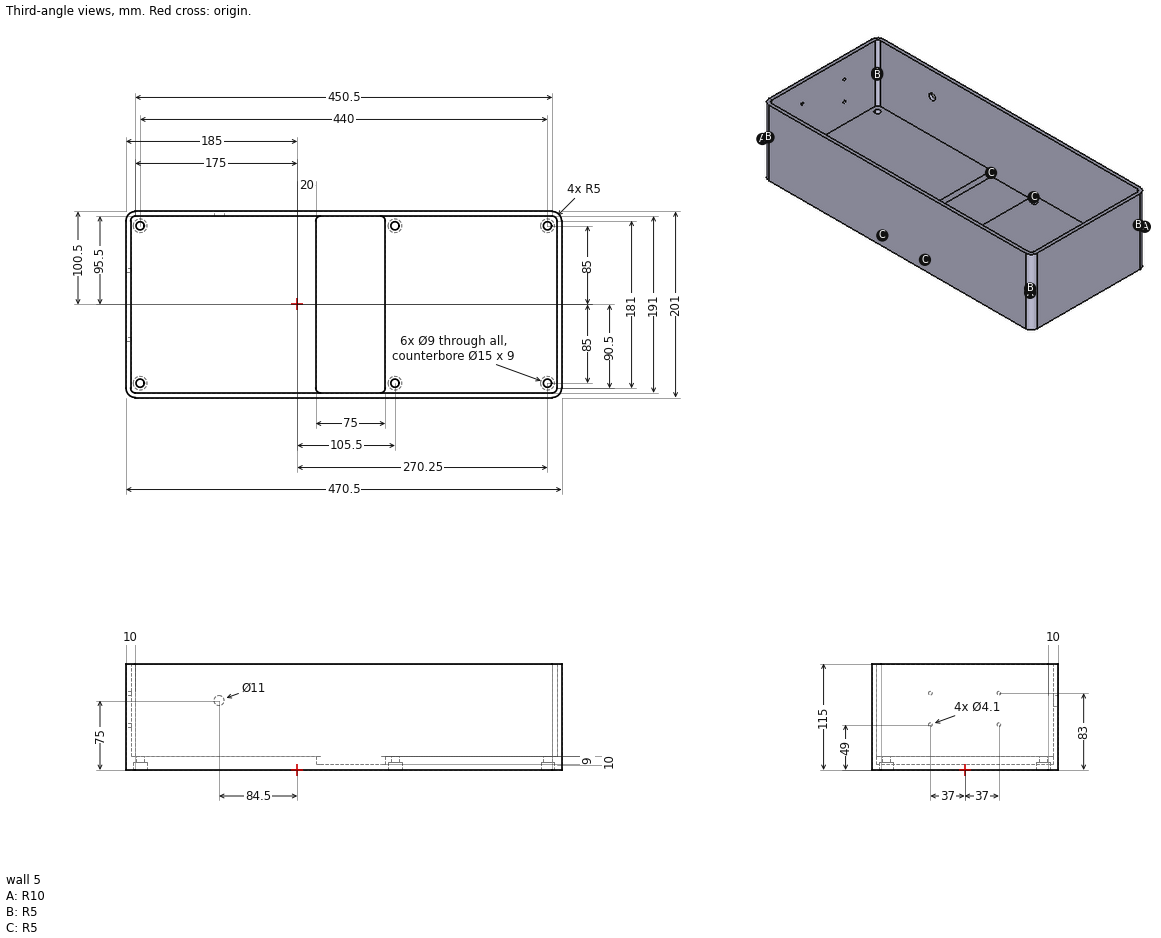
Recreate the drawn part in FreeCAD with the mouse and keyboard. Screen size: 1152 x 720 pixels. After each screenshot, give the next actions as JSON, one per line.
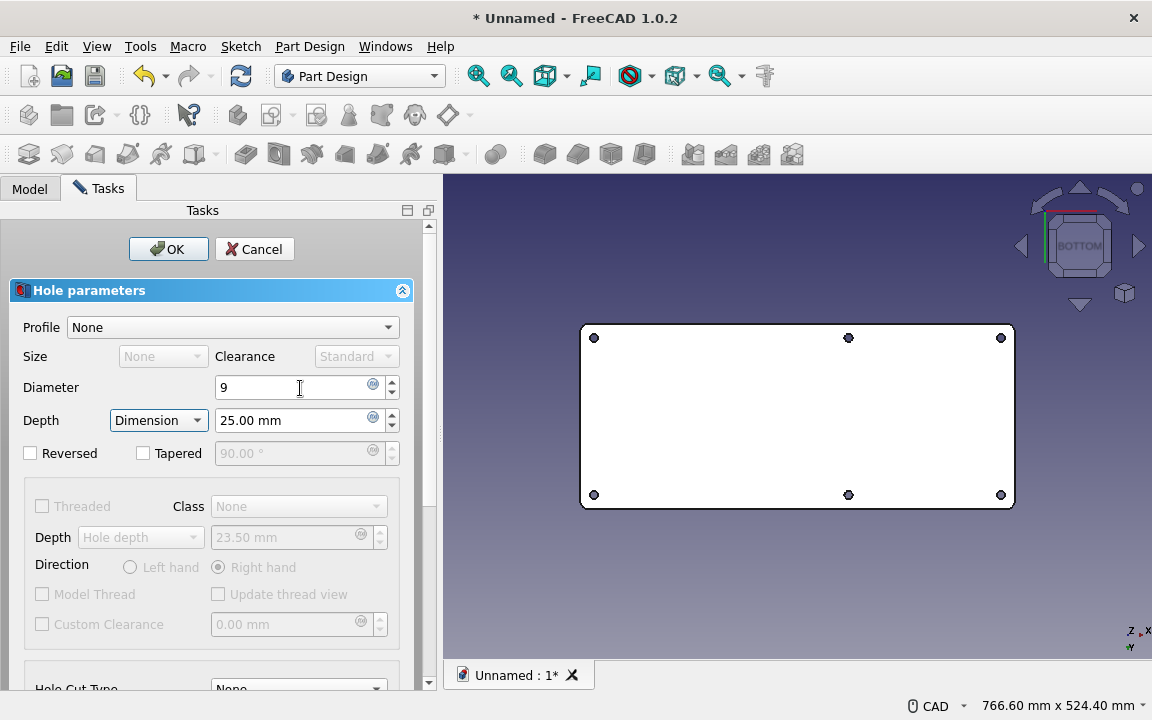
{"action": "left_click", "coordinate": [160, 420]}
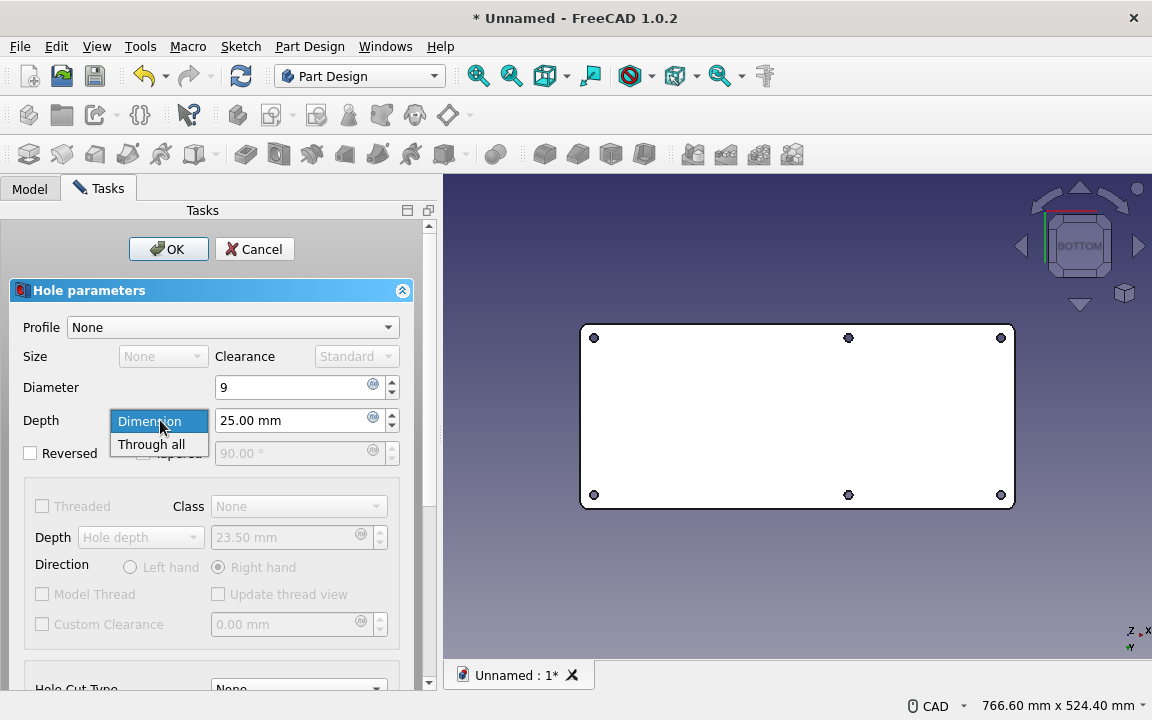
{"action": "left_click", "coordinate": [158, 444]}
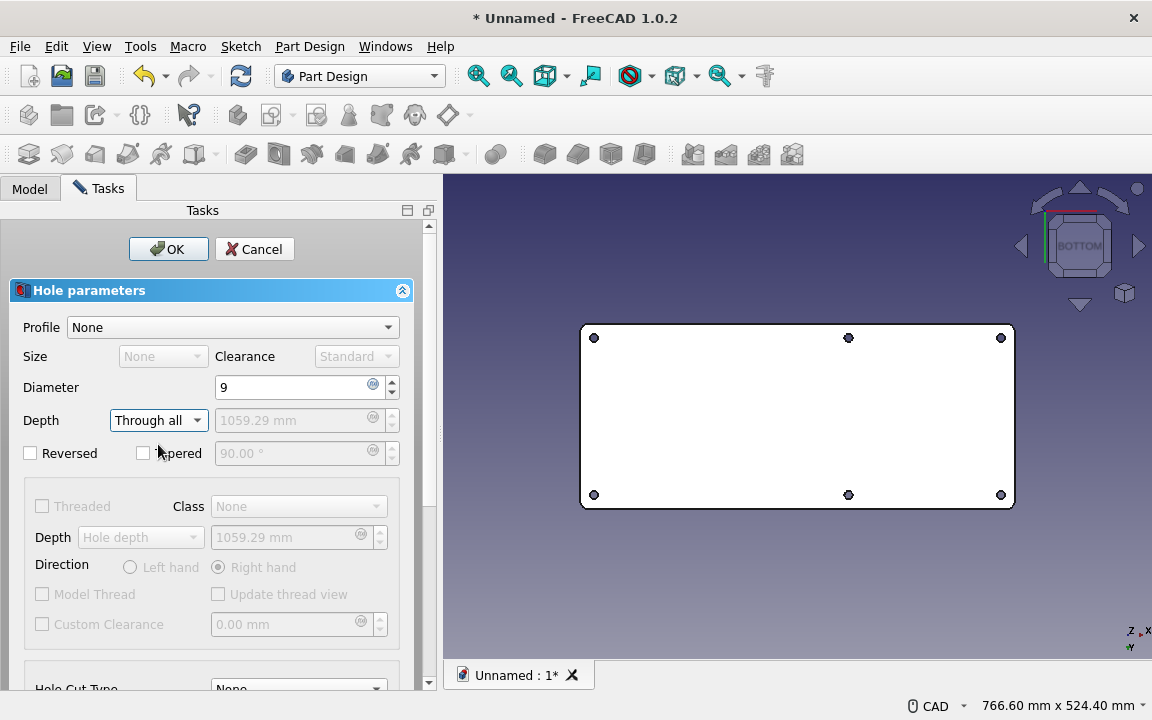
{"action": "scroll", "coordinate": [429, 455], "scroll_direction": "down", "scroll_amount": 2}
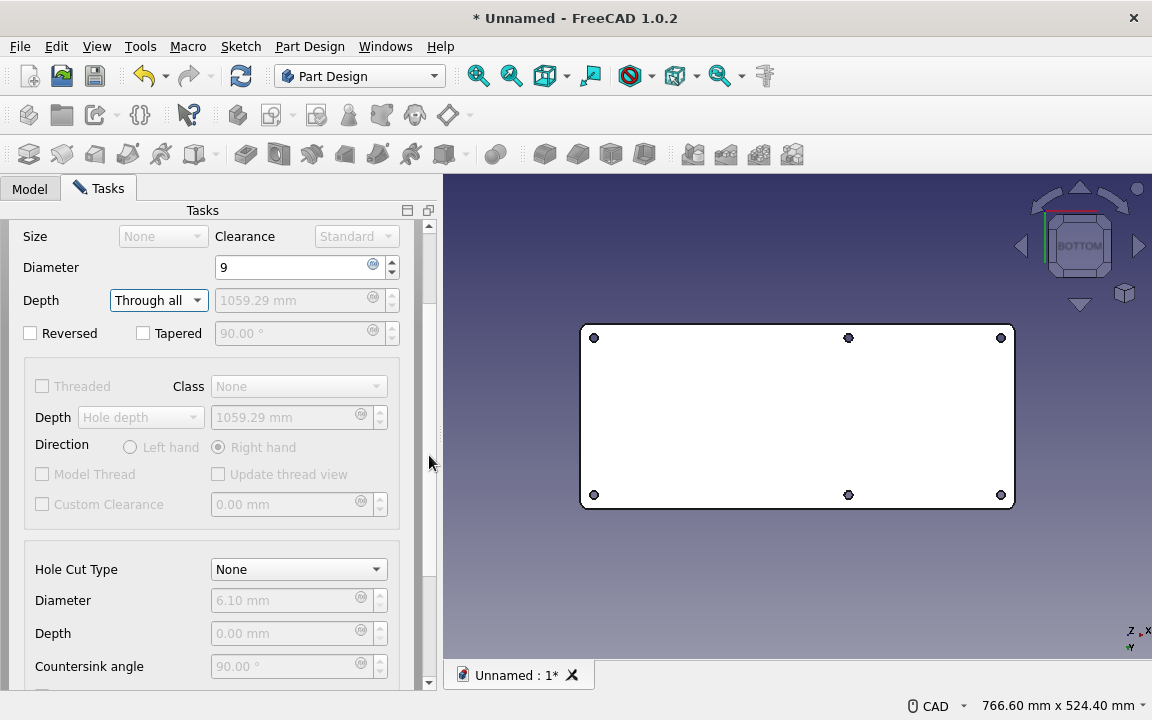
{"action": "left_click", "coordinate": [300, 570]}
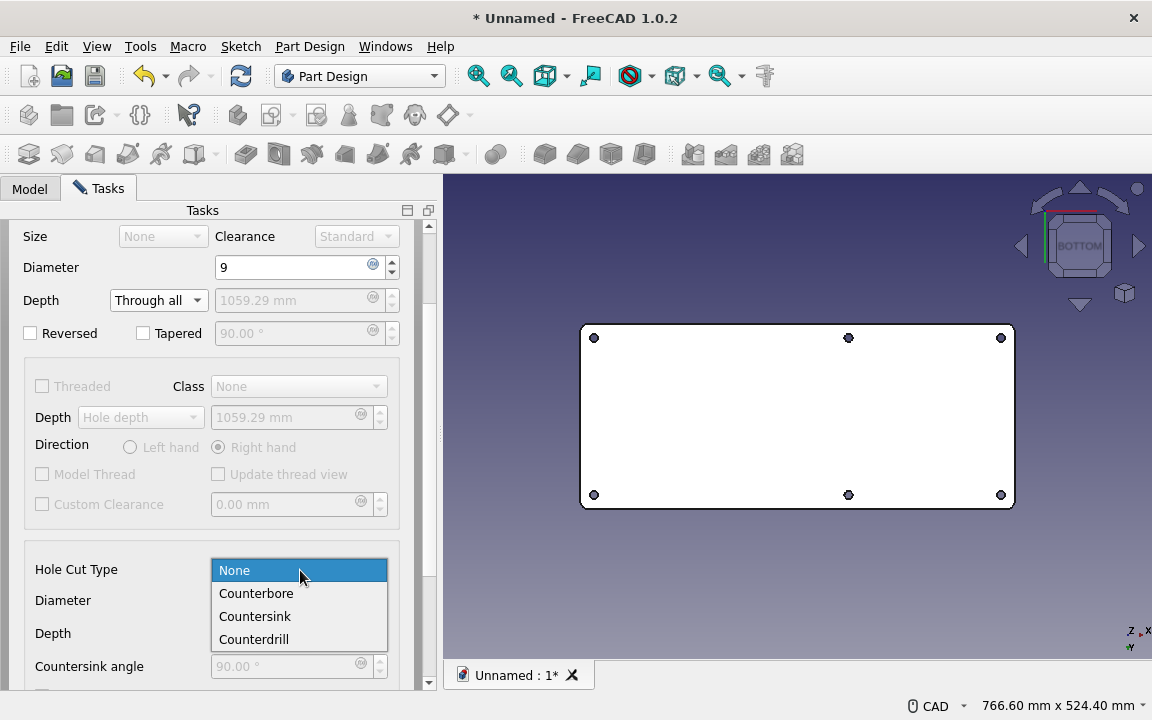
{"action": "left_click", "coordinate": [298, 594]}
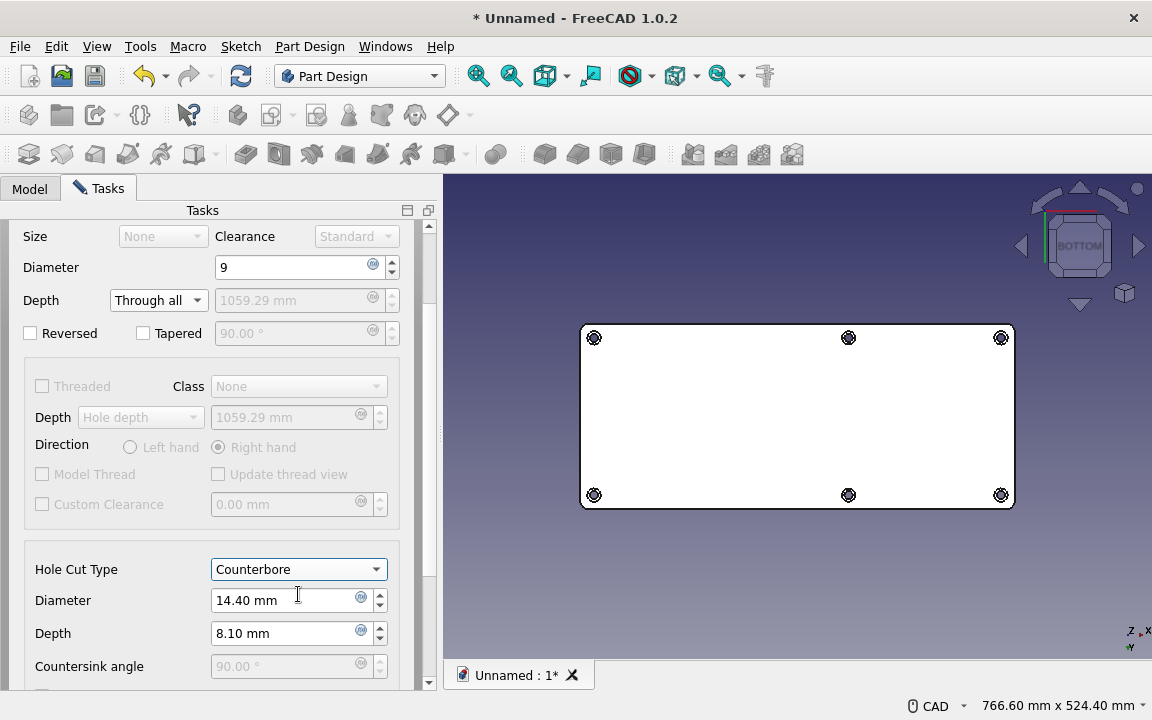
{"action": "triple_click", "coordinate": [292, 600]}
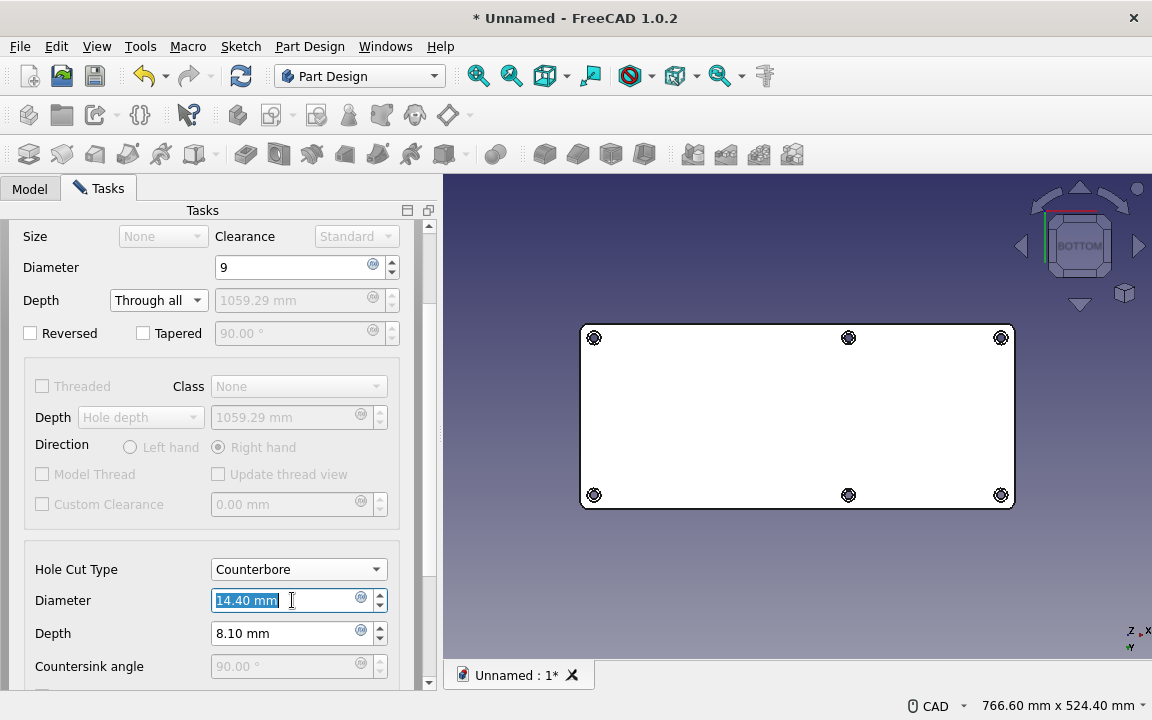
{"action": "type", "text": "15"}
{"action": "key", "text": "Tab"}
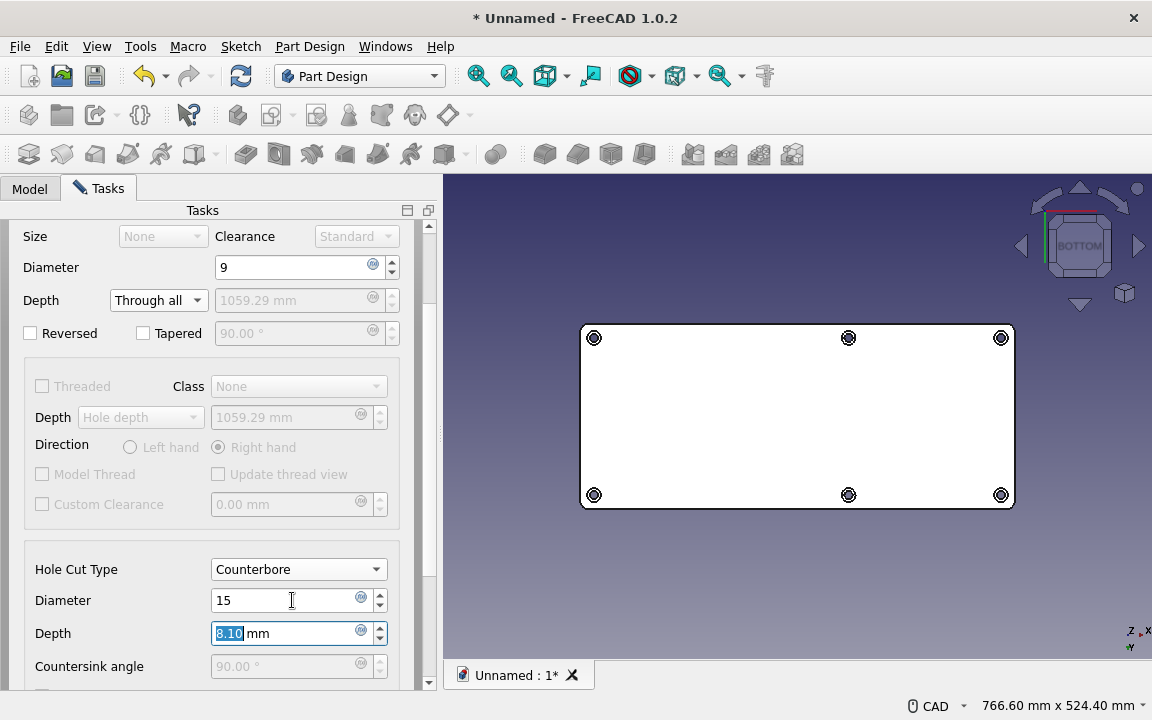
{"action": "type", "text": "9"}
{"action": "key", "text": "Tab"}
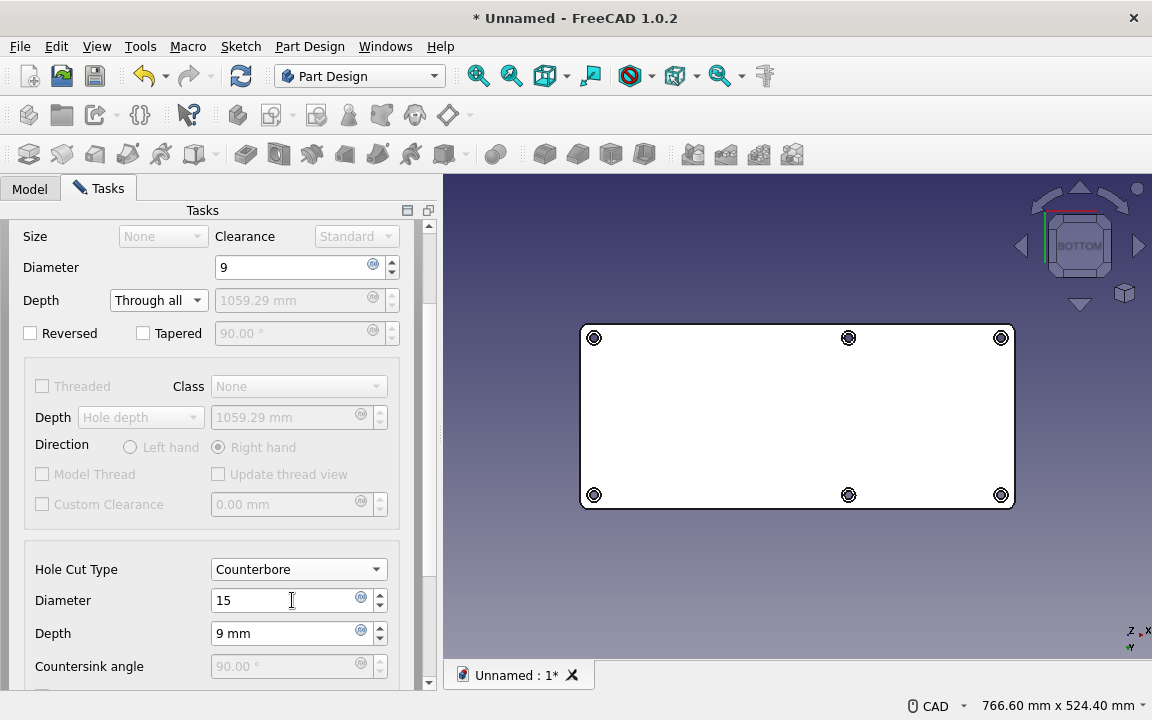
{"action": "scroll", "coordinate": [429, 455], "scroll_direction": "up", "scroll_amount": 3}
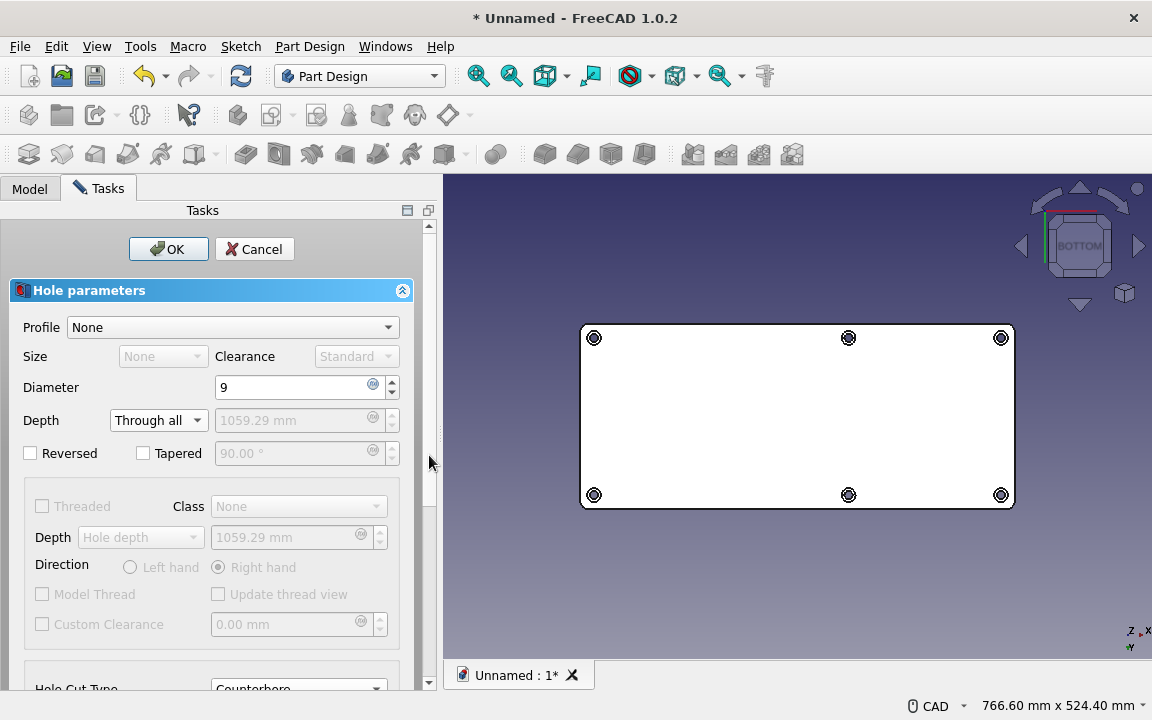
{"action": "left_click", "coordinate": [169, 249]}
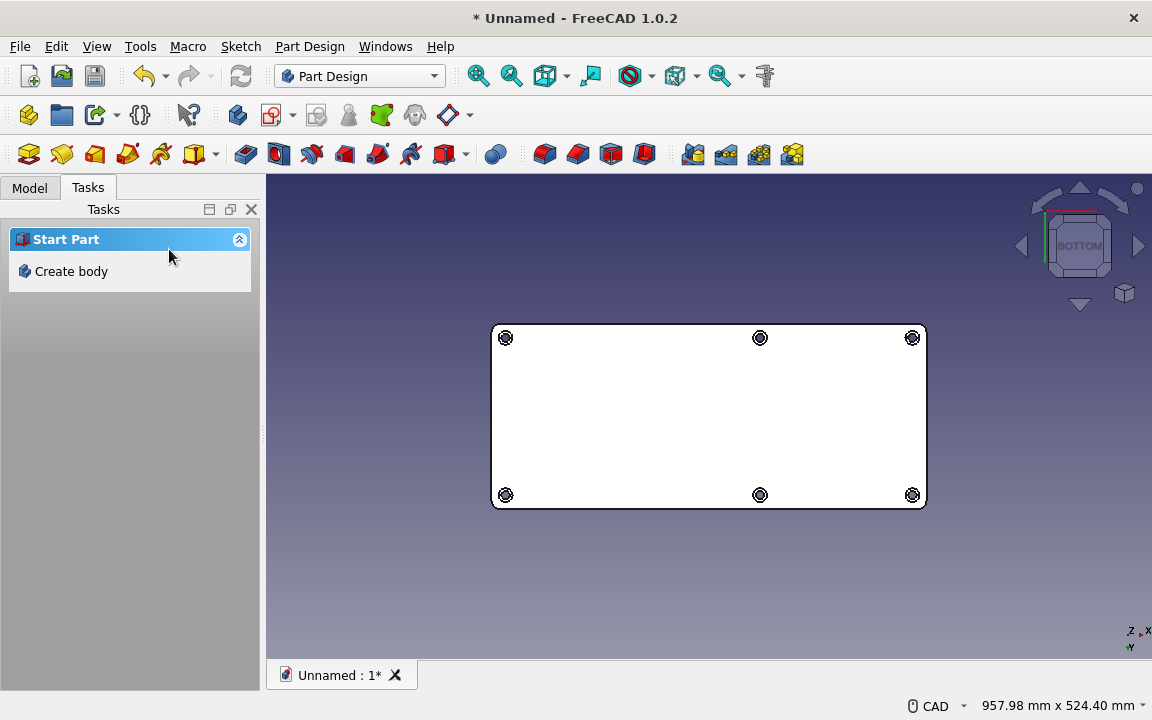
{"action": "key", "text": "0"}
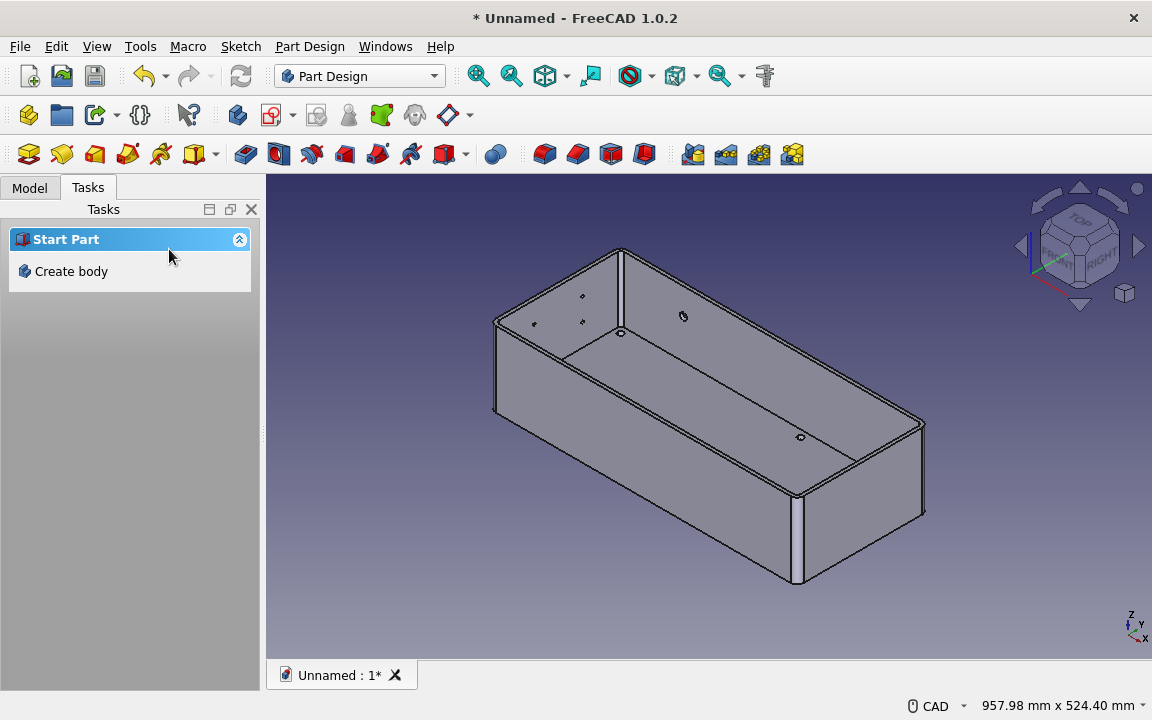
{"action": "left_click", "coordinate": [727, 437]}